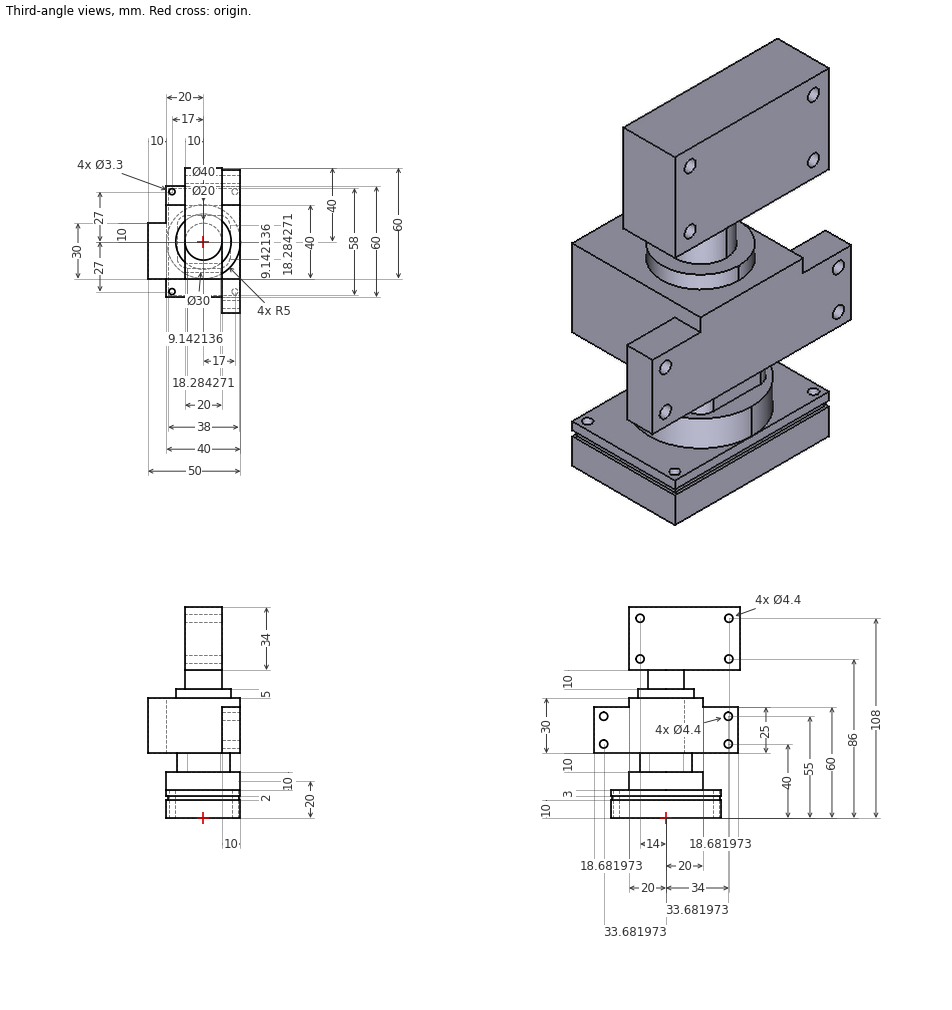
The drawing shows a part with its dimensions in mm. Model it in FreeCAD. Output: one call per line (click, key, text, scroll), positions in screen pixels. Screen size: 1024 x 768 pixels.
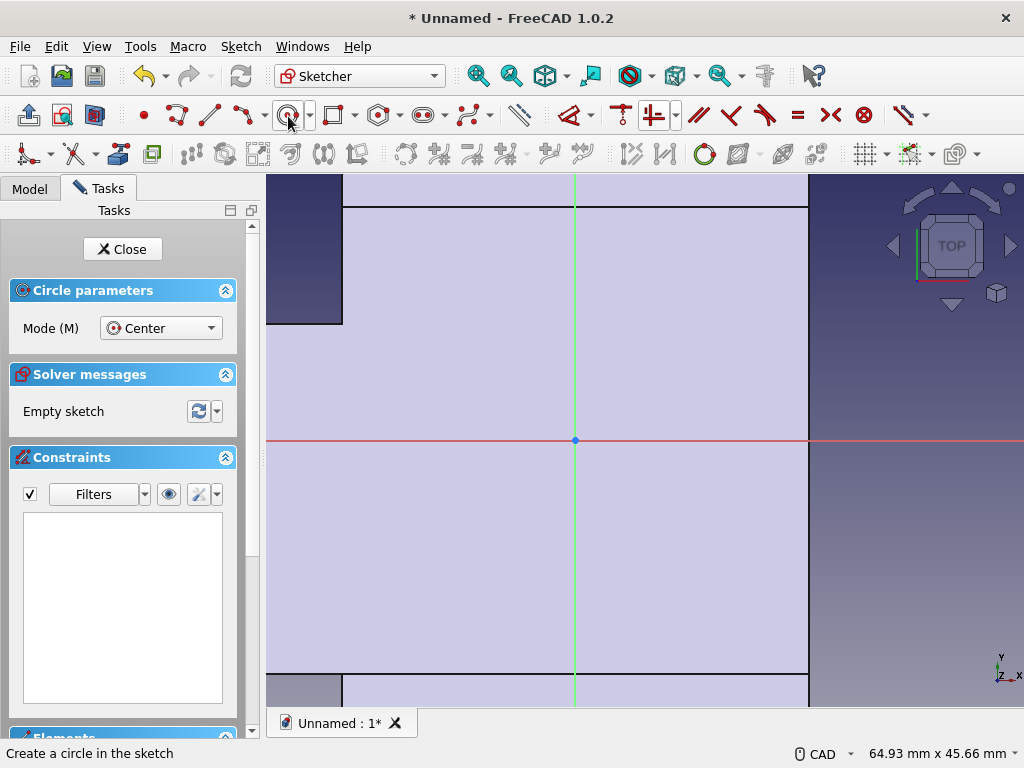
click(575, 440)
move(699, 317)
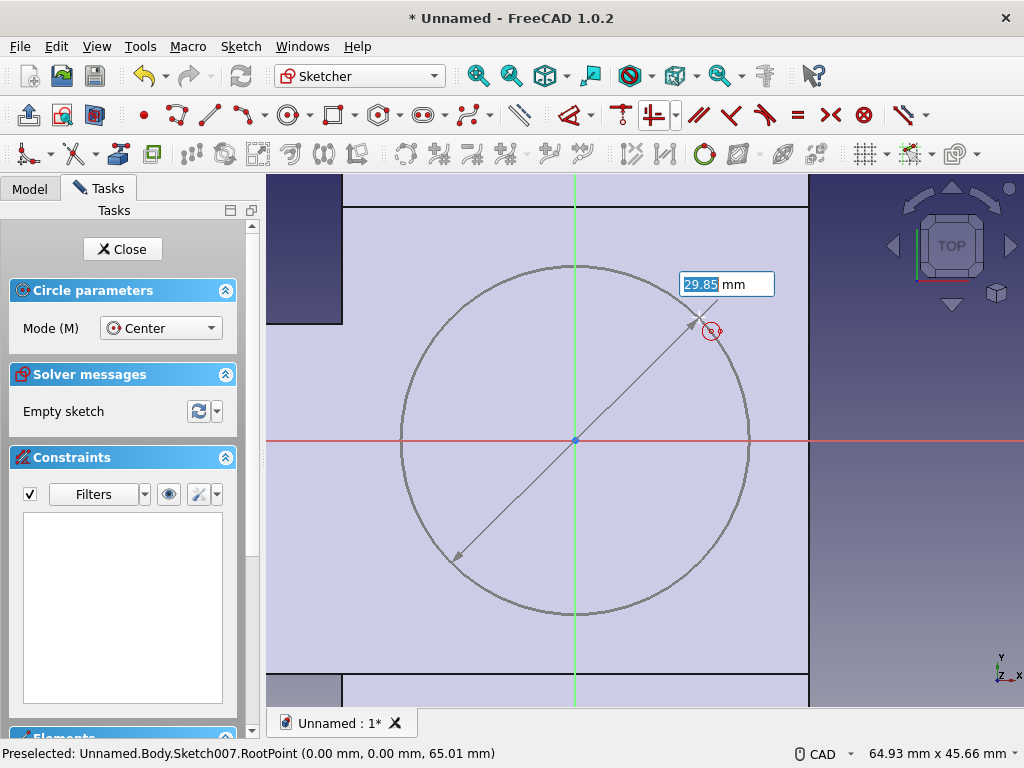
text(30)
key(Return)
key(Escape)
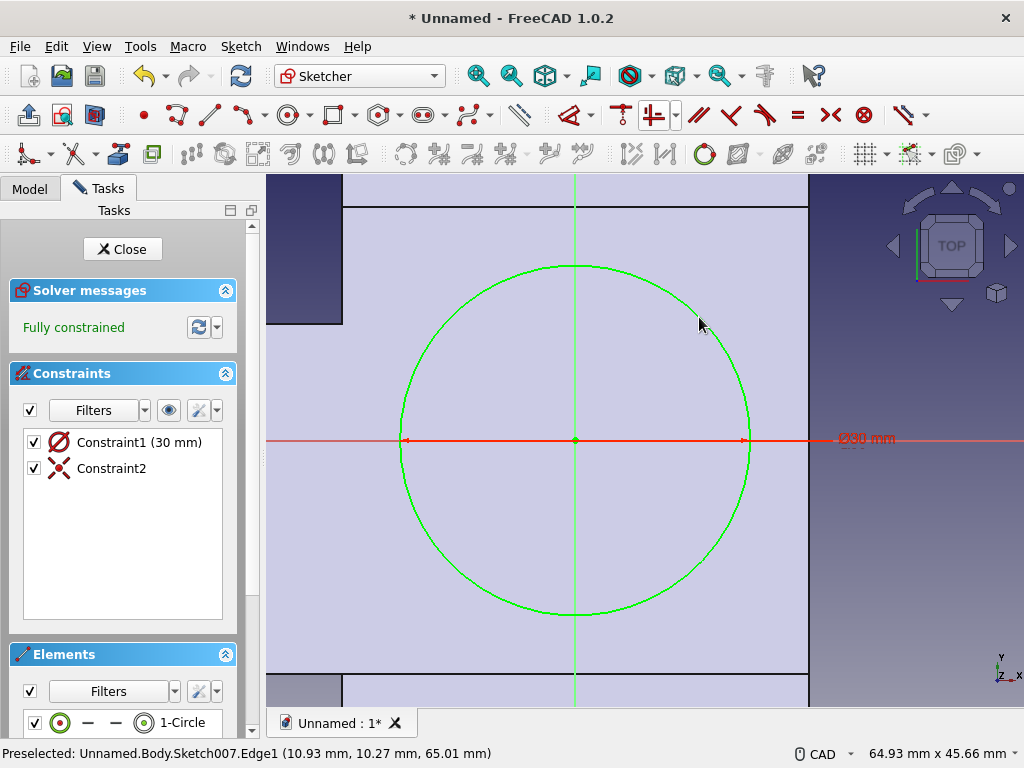
click(123, 249)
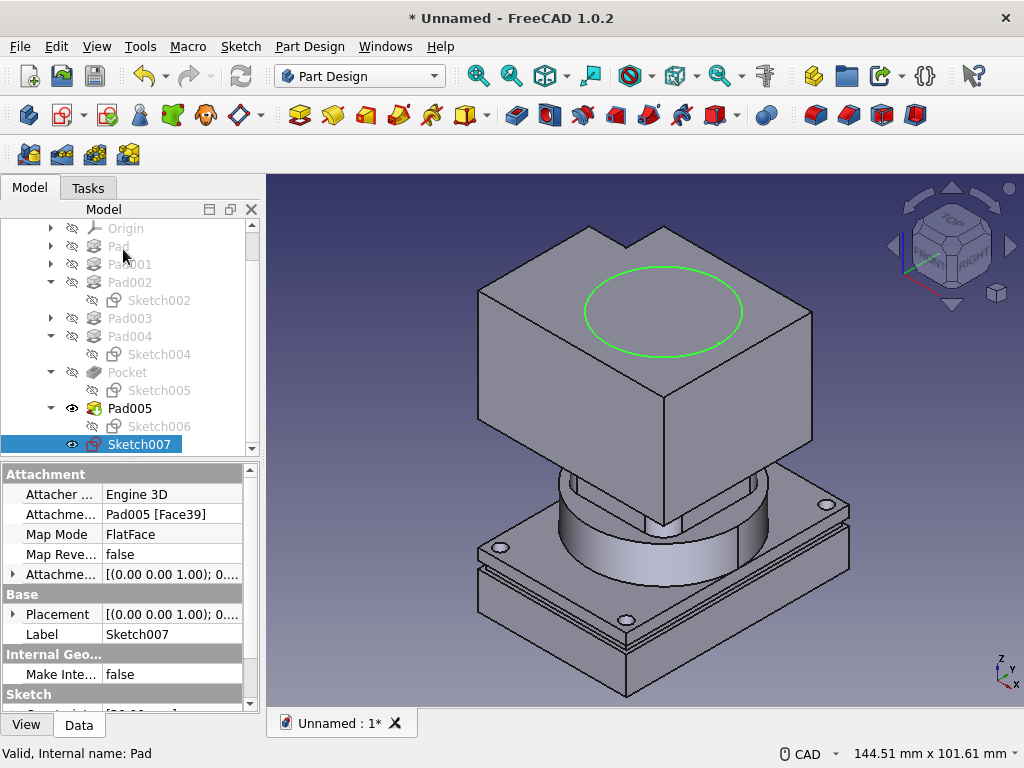
click(300, 116)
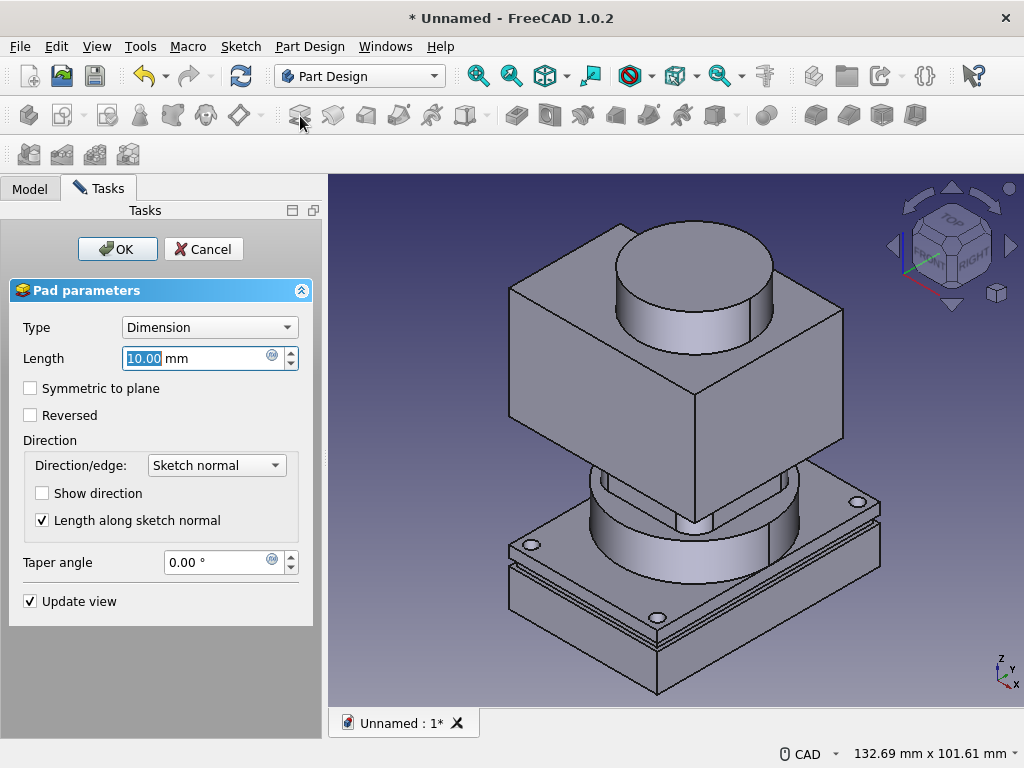
text(5)
key(Tab)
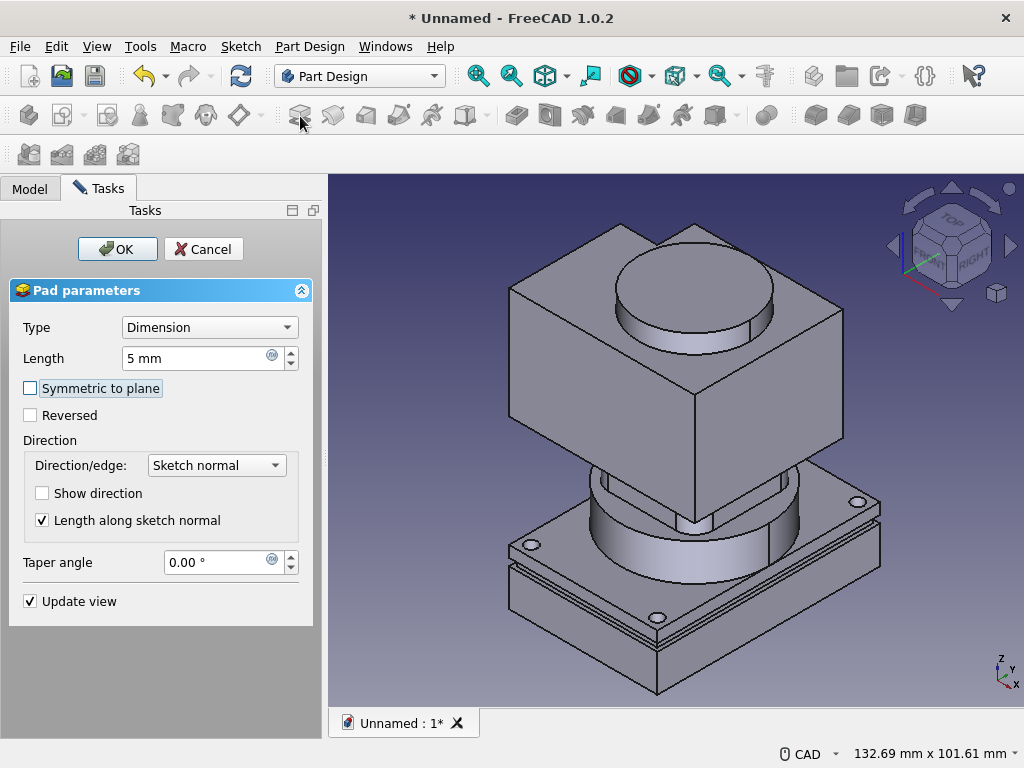
click(118, 249)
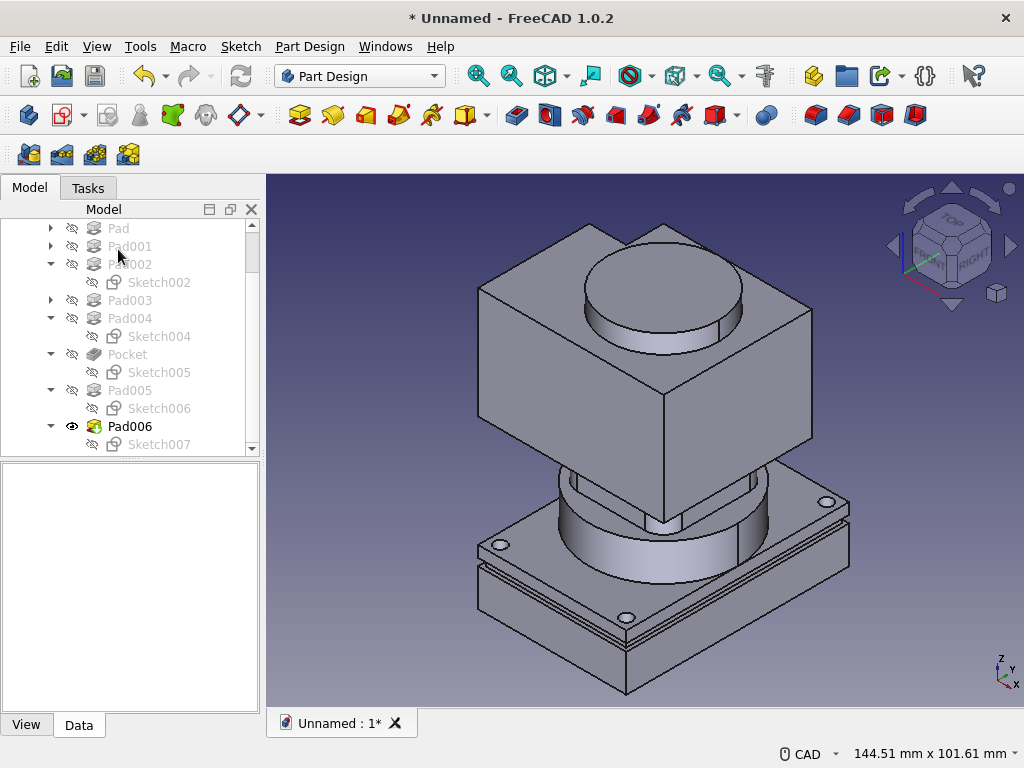
key(v)
key(f)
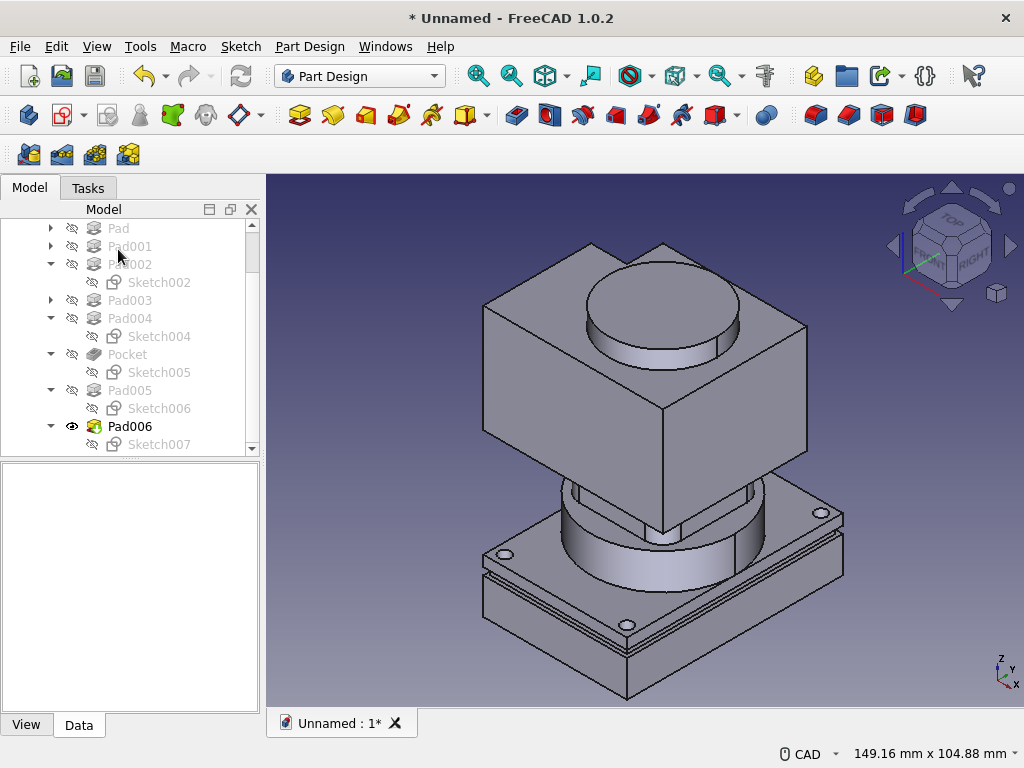
click(663, 305)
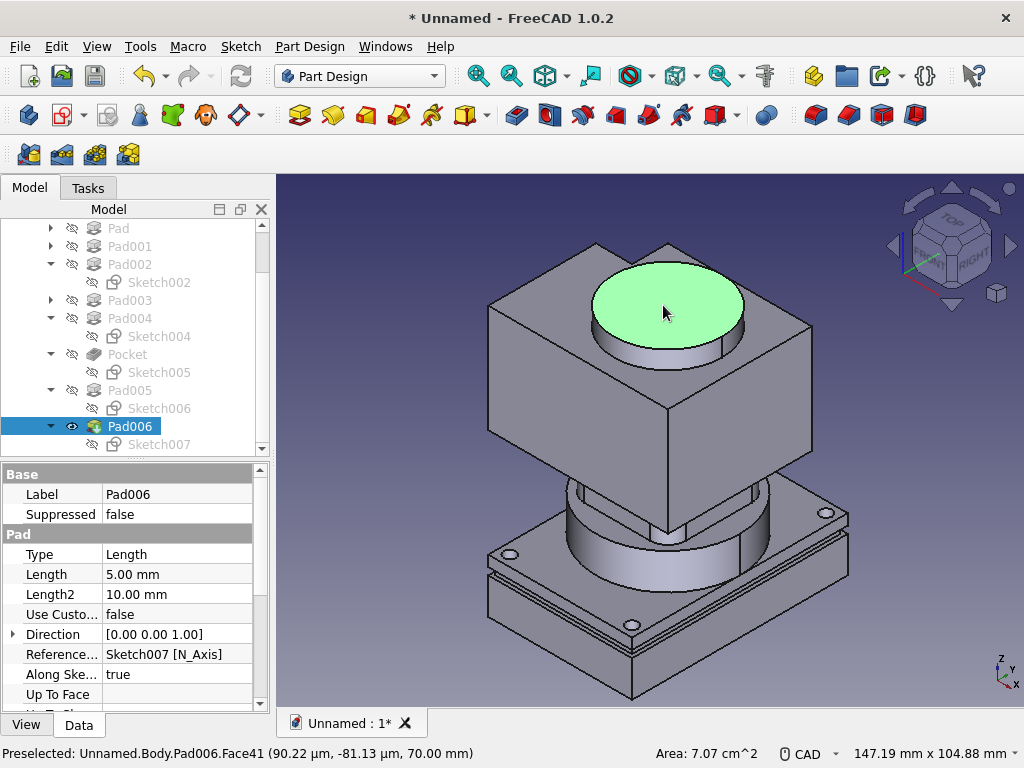
click(62, 116)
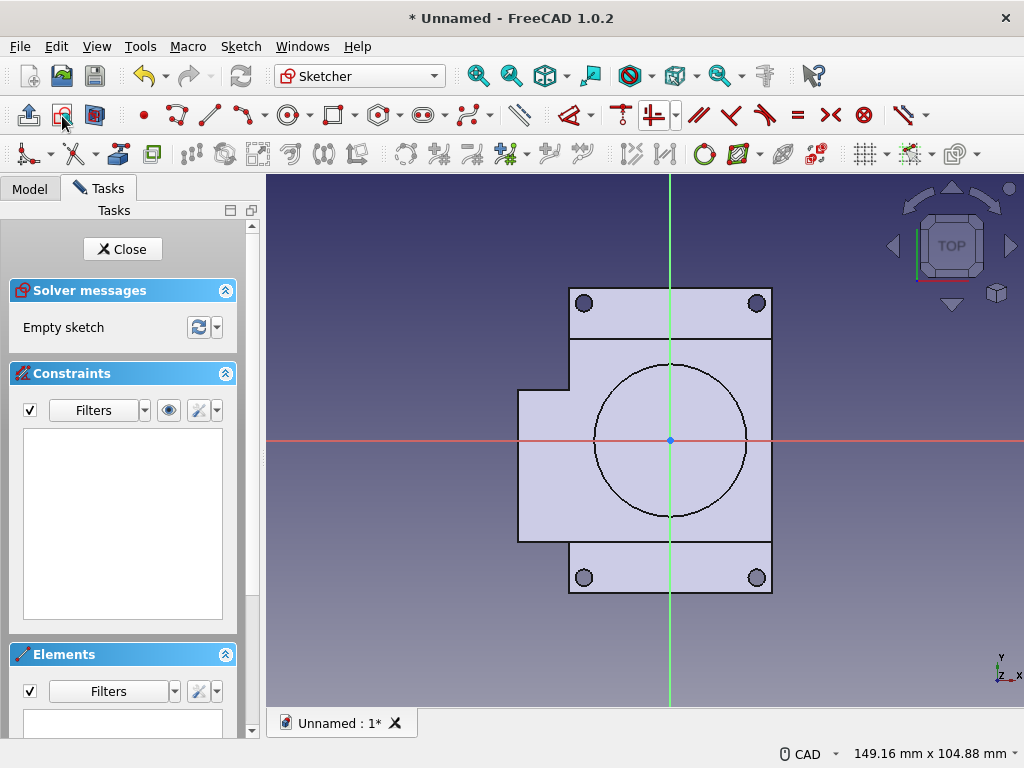
scroll(711, 440, up, 6)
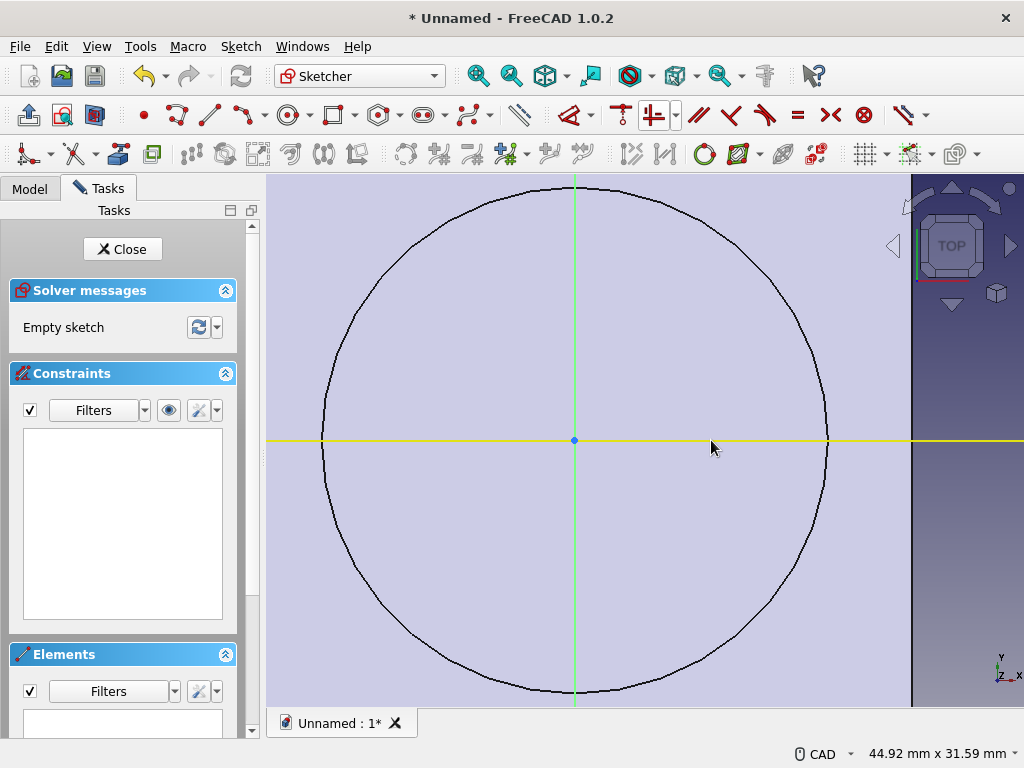
key(g)
key(c)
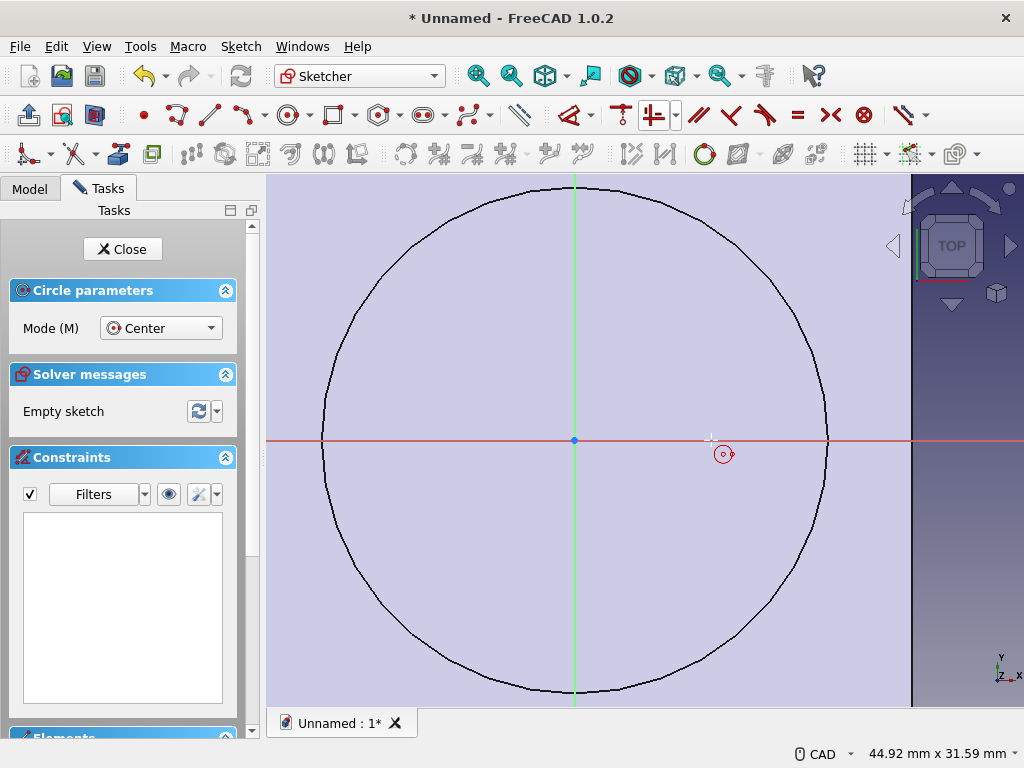
click(575, 440)
move(694, 321)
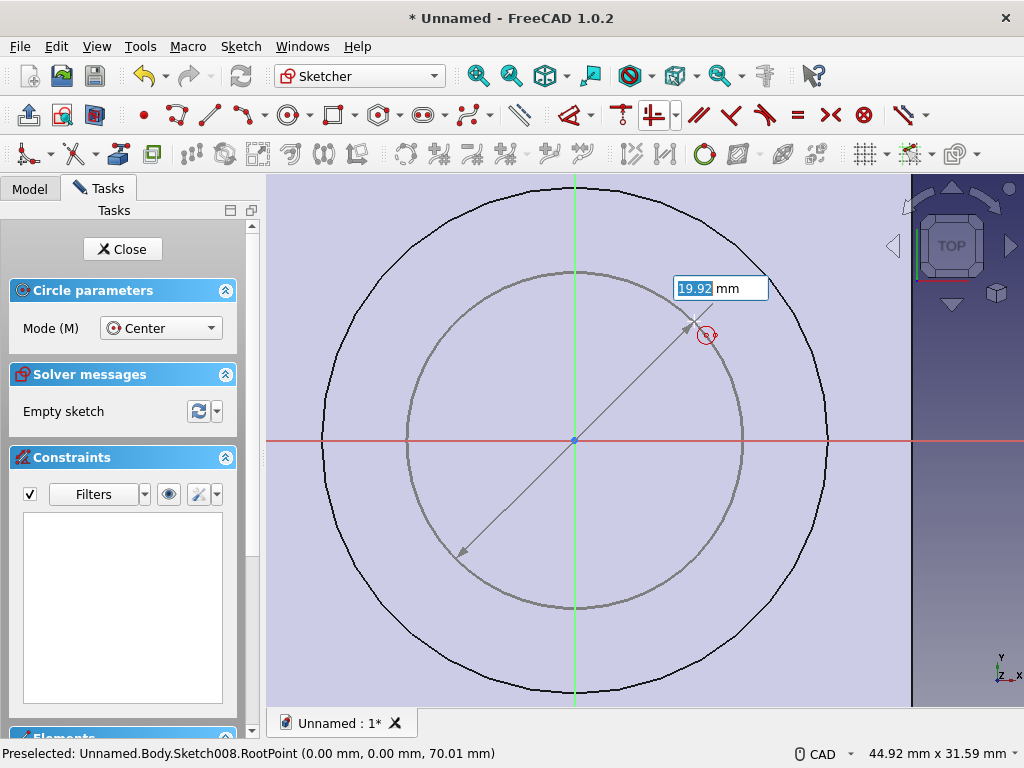
text(20)
key(Return)
key(Escape)